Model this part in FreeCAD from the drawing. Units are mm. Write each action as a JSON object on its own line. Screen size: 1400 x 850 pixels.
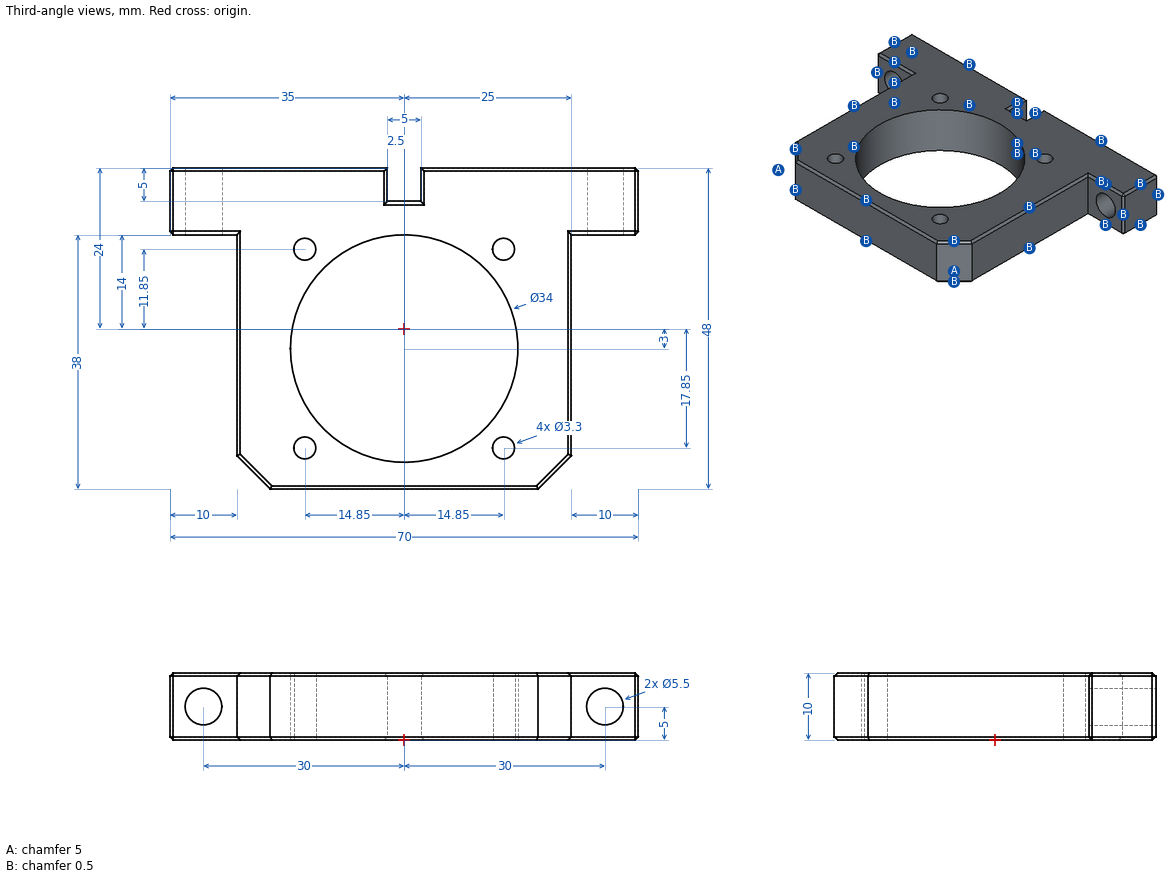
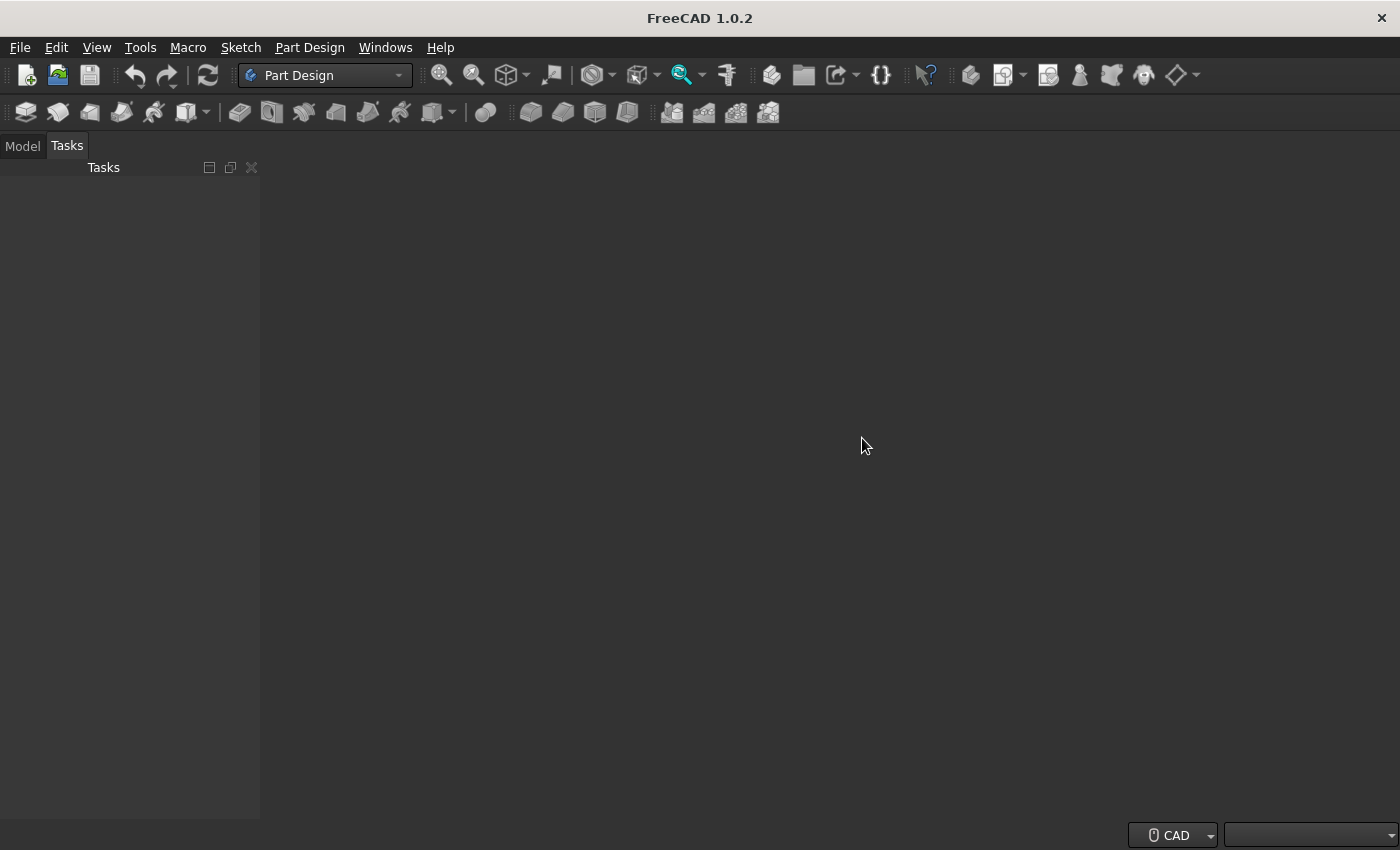
{"action": "left_click", "coordinate": [26, 76]}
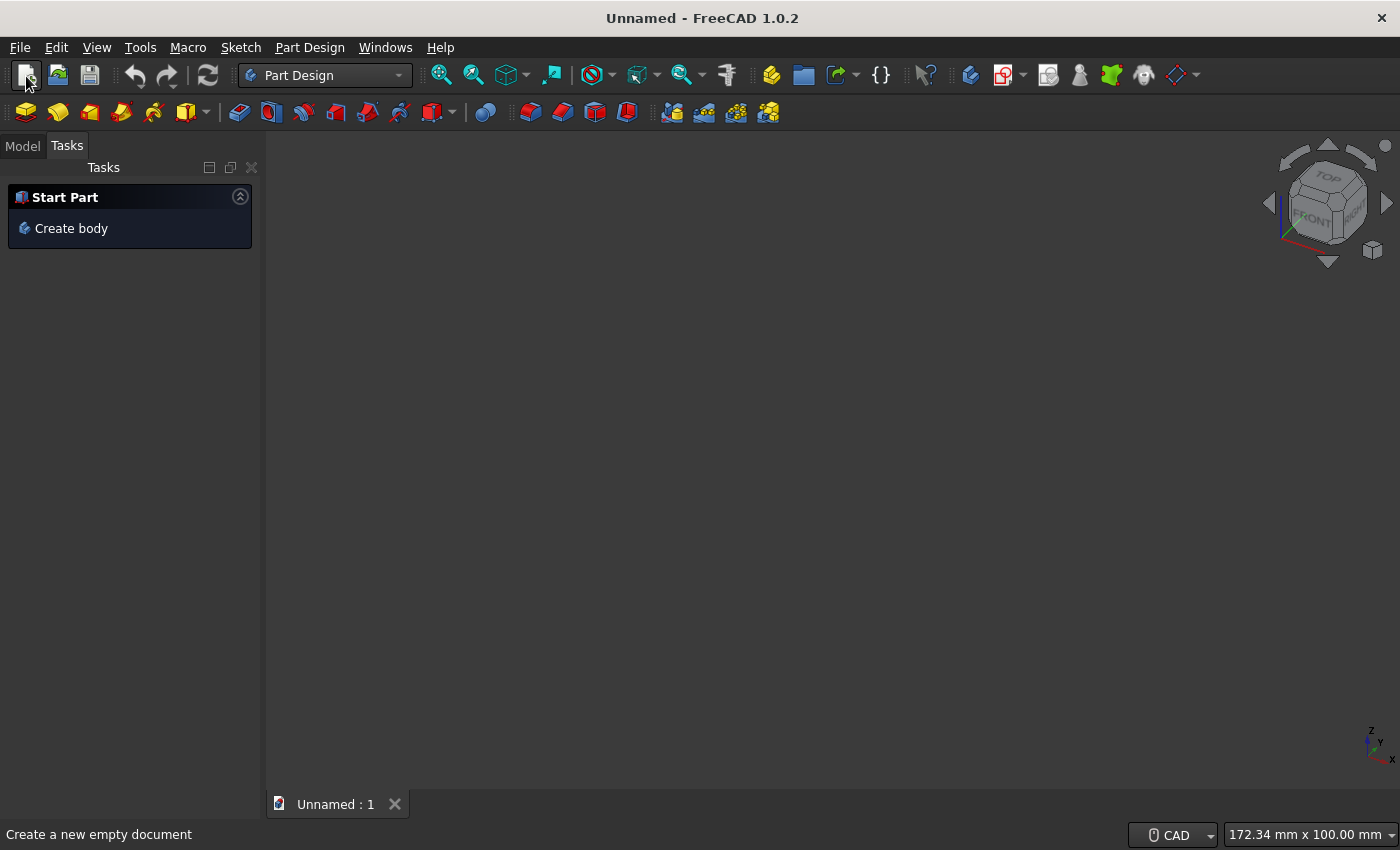
{"action": "left_click", "coordinate": [1004, 76]}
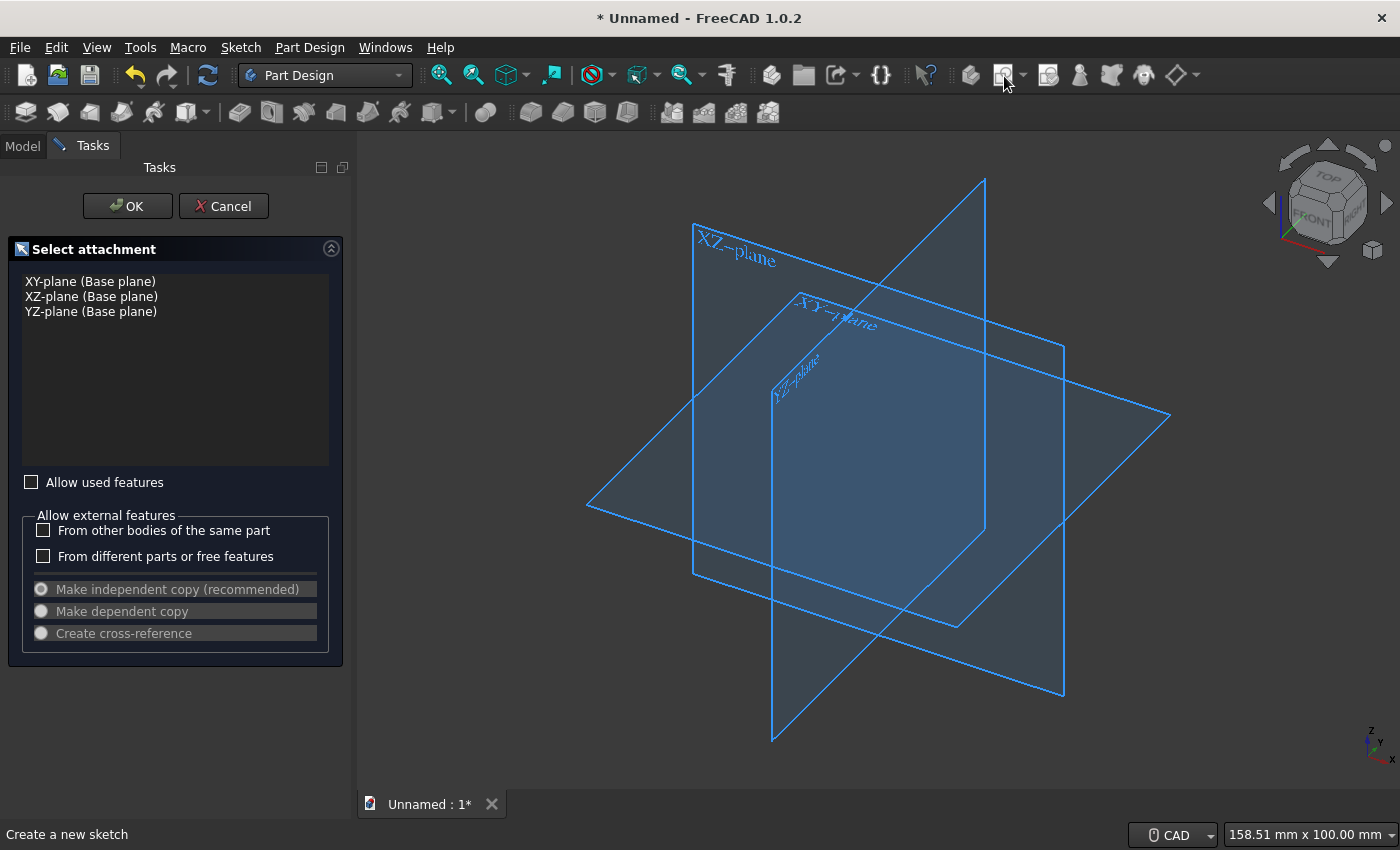
{"action": "left_click", "coordinate": [82, 282]}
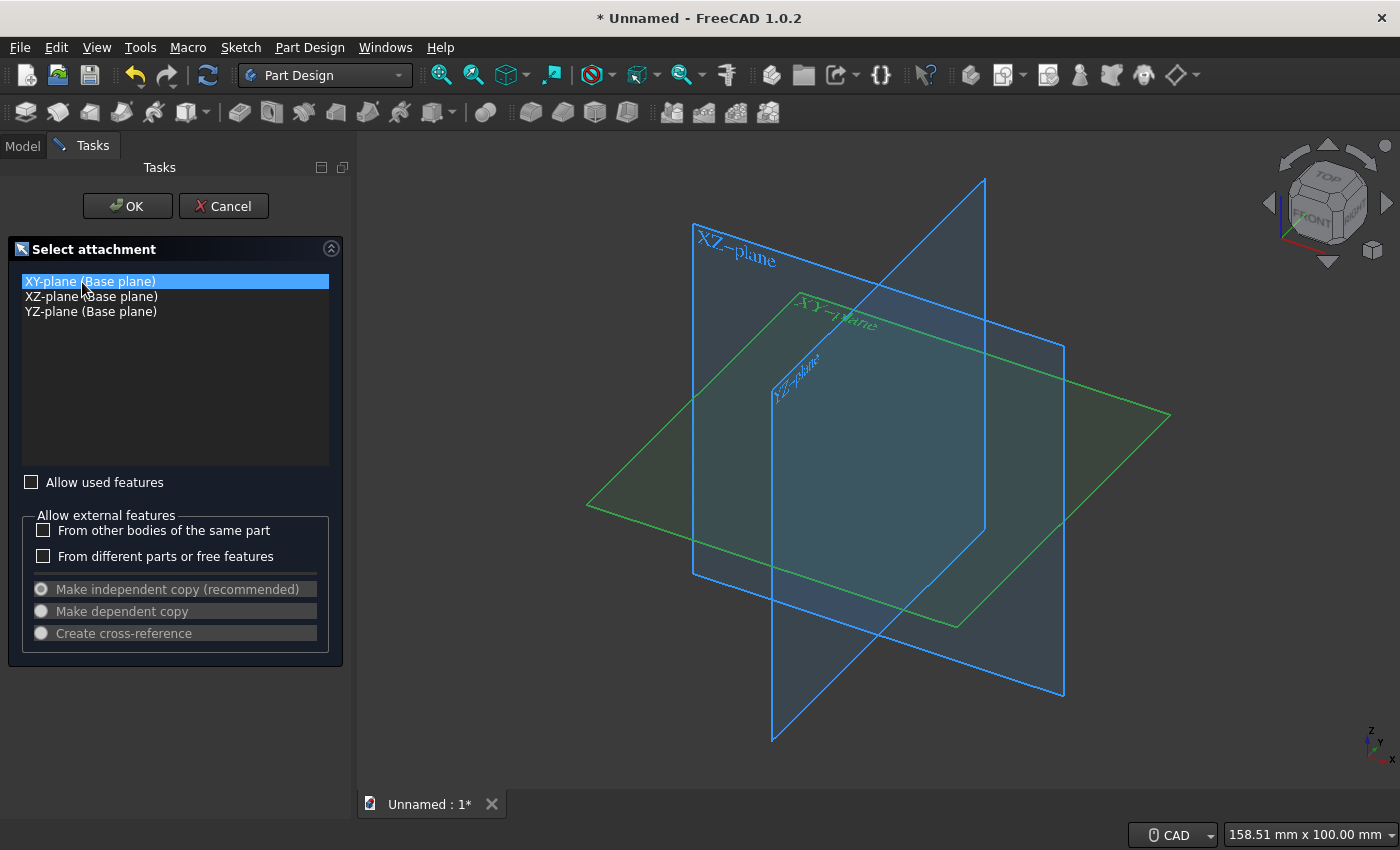
{"action": "left_click", "coordinate": [128, 206]}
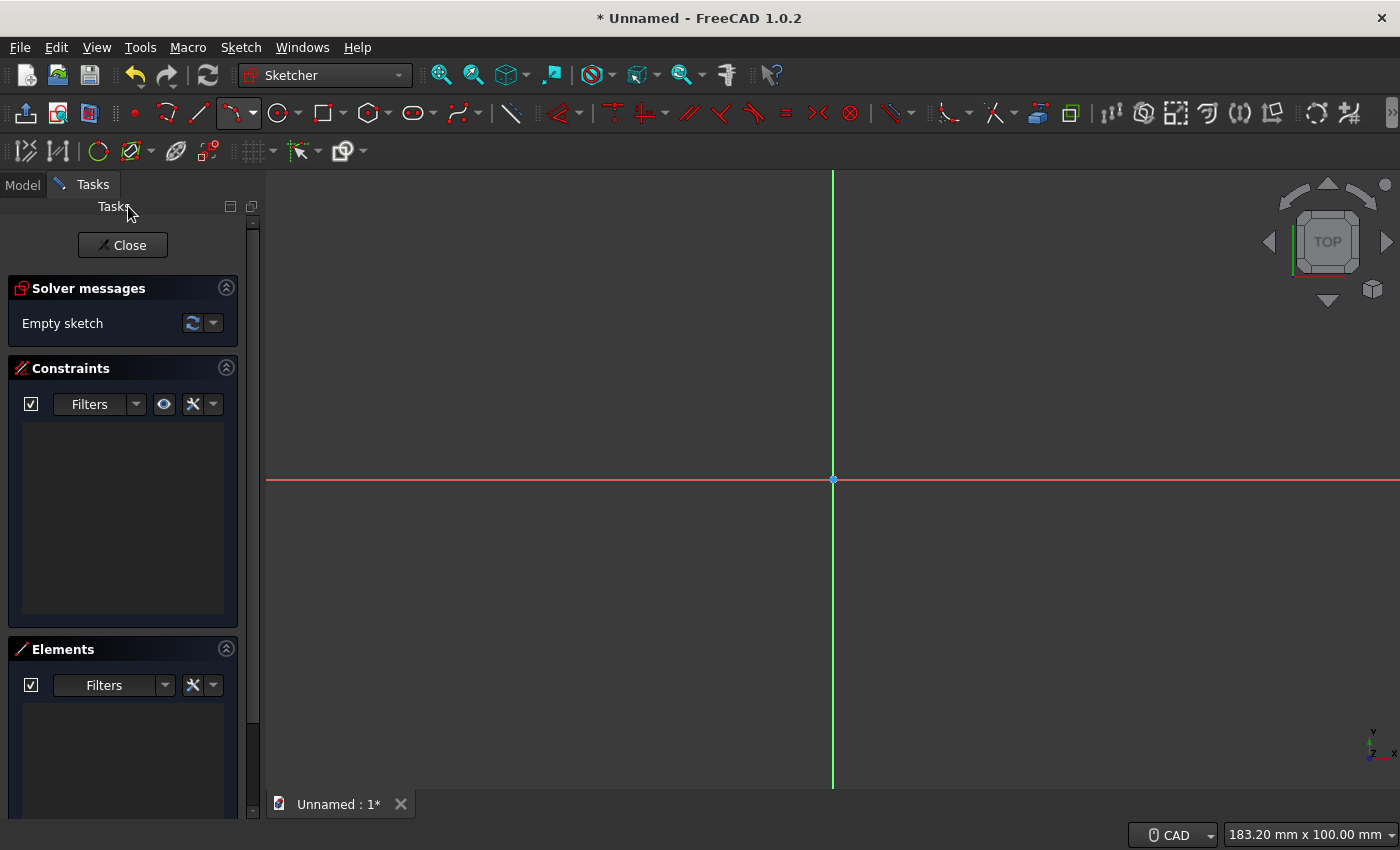
{"action": "left_click", "coordinate": [346, 114]}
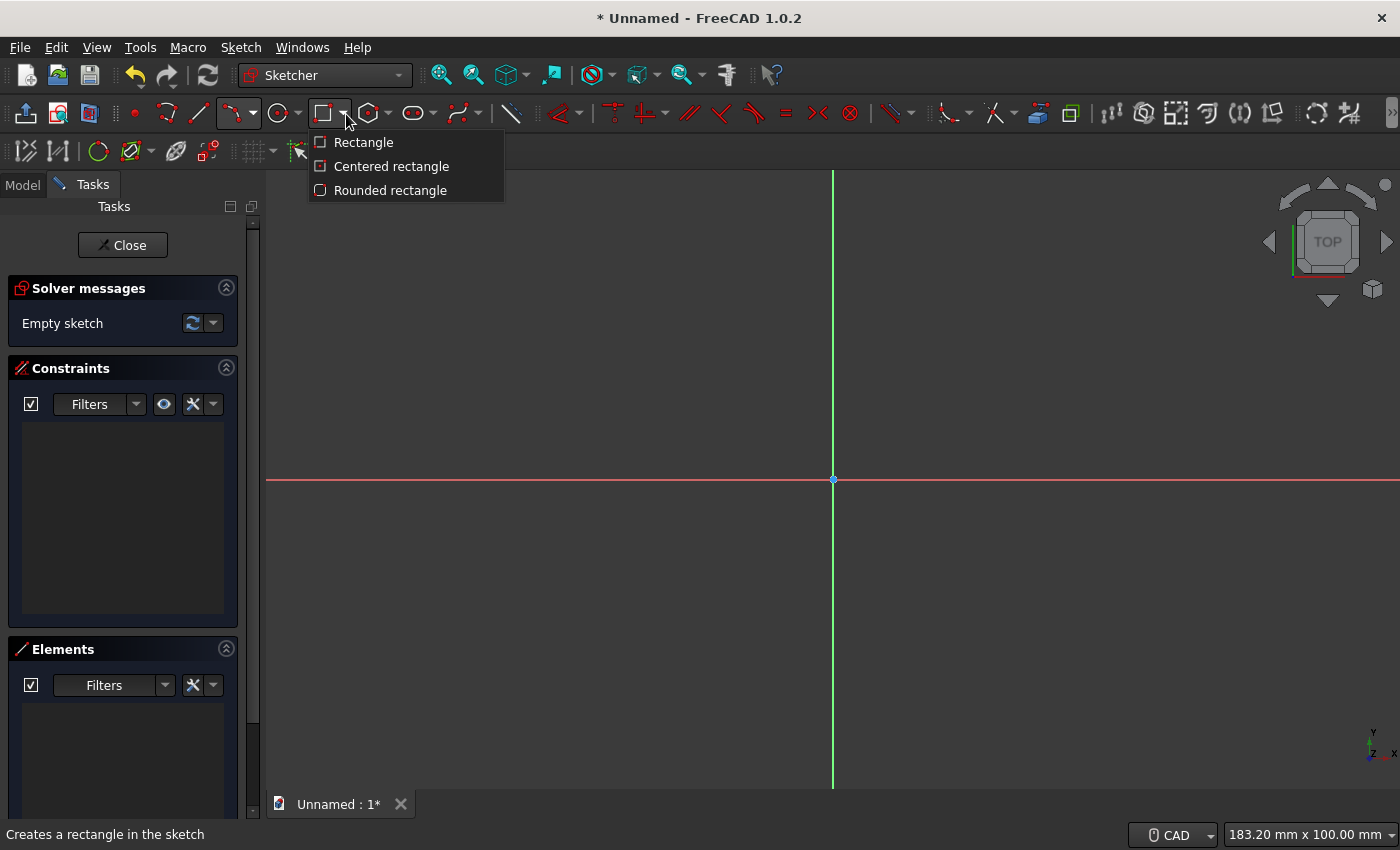
{"action": "left_click", "coordinate": [406, 166]}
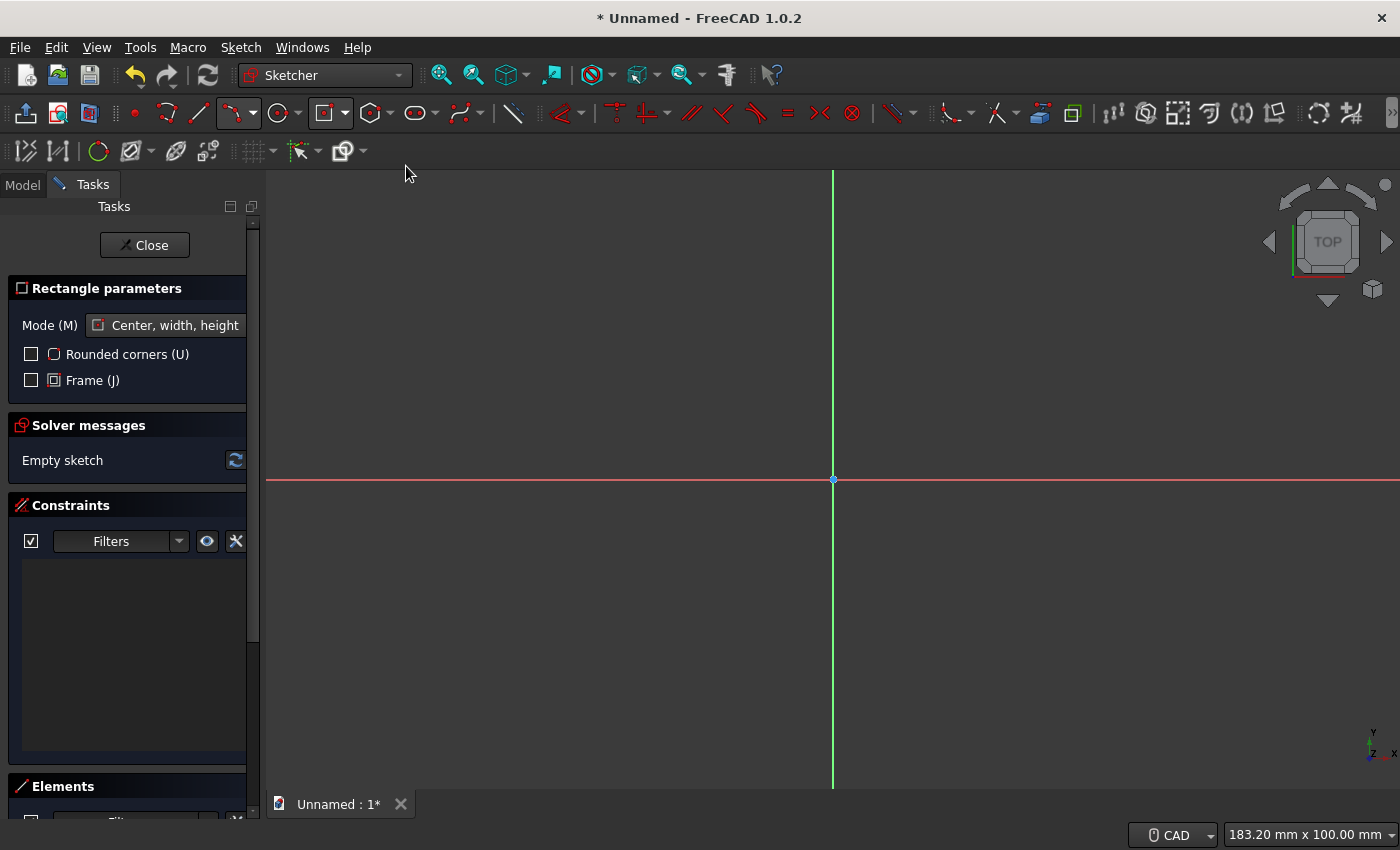
{"action": "left_click", "coordinate": [833, 480]}
{"action": "left_click", "coordinate": [1050, 331]}
{"action": "key", "text": "Escape"}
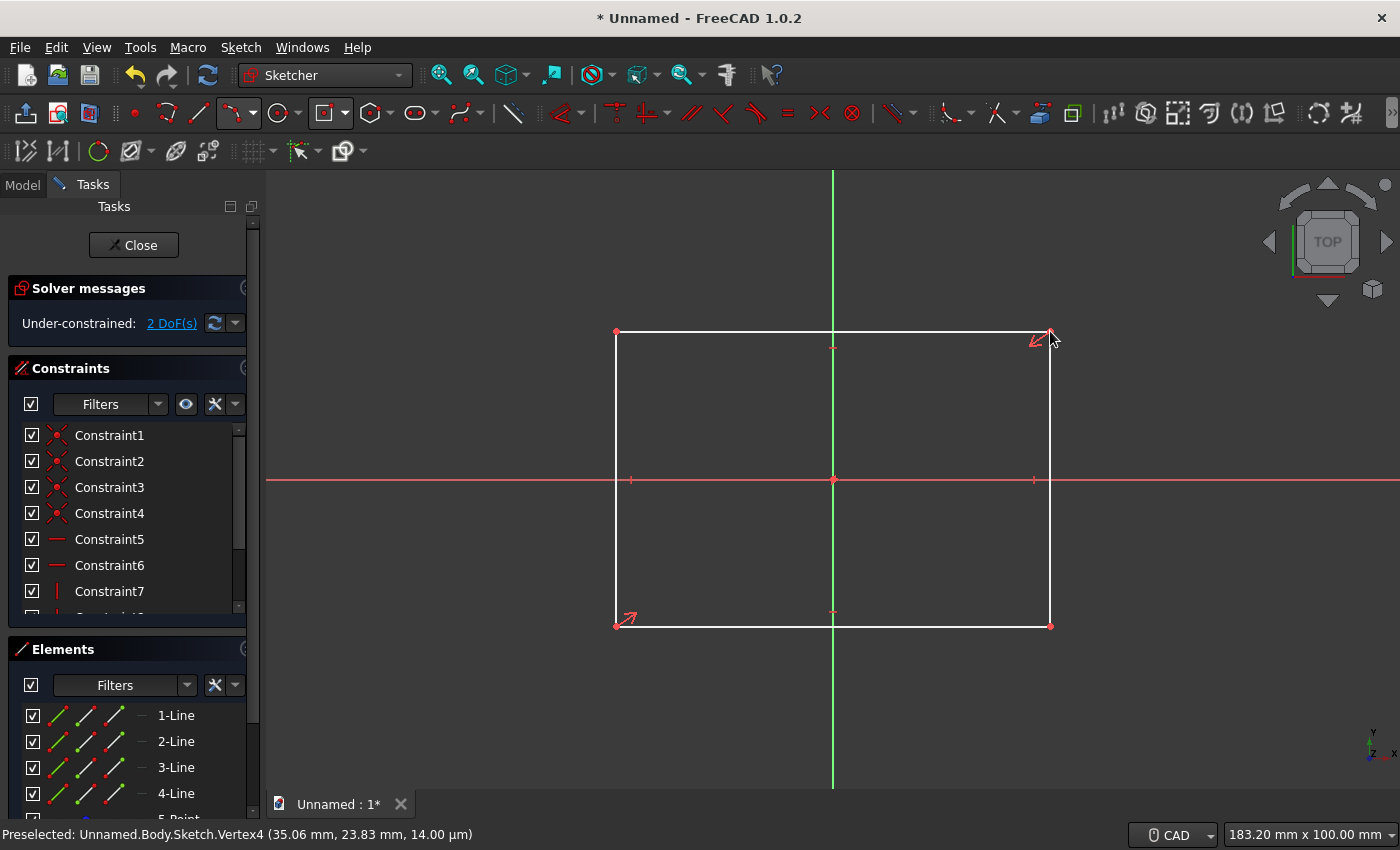
{"action": "left_click", "coordinate": [746, 627]}